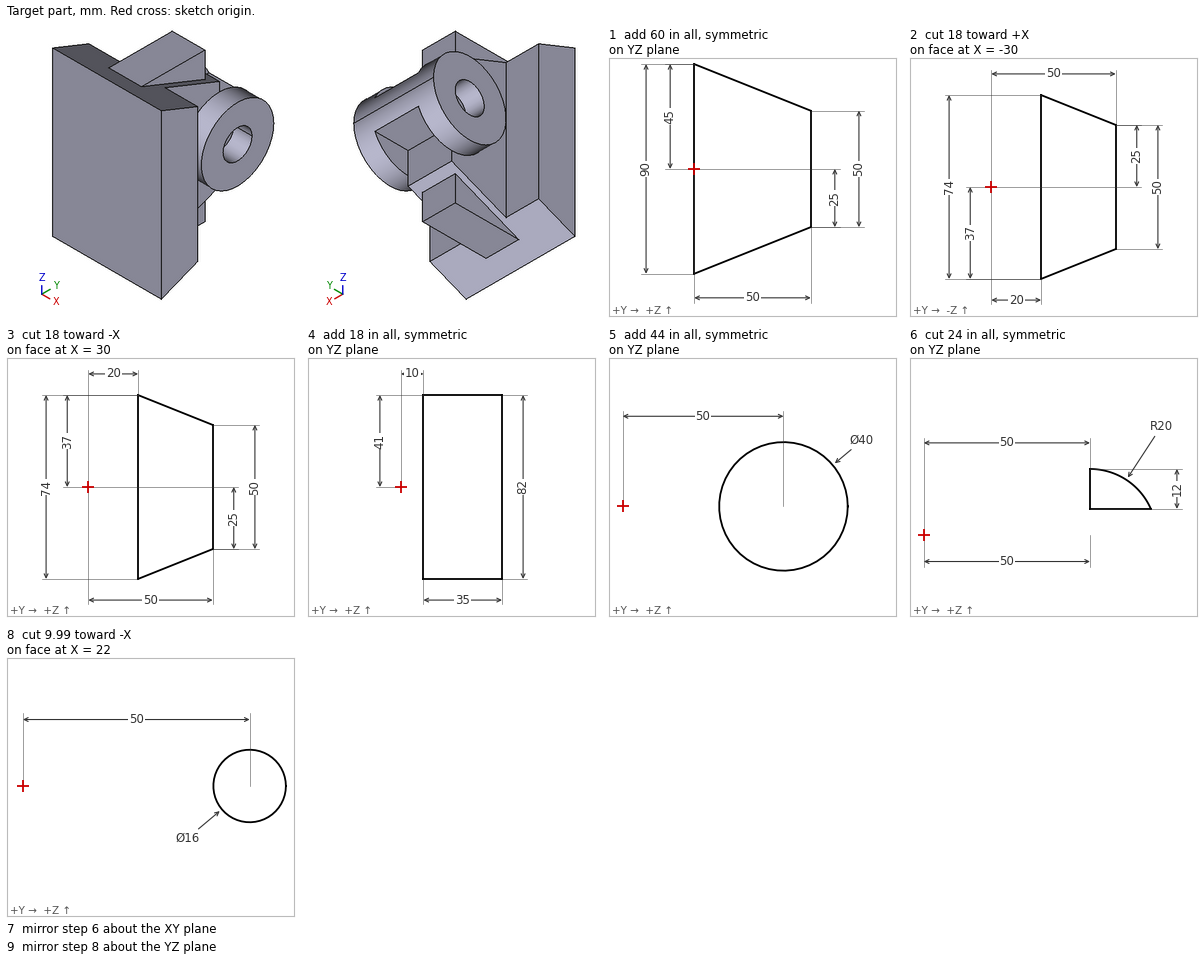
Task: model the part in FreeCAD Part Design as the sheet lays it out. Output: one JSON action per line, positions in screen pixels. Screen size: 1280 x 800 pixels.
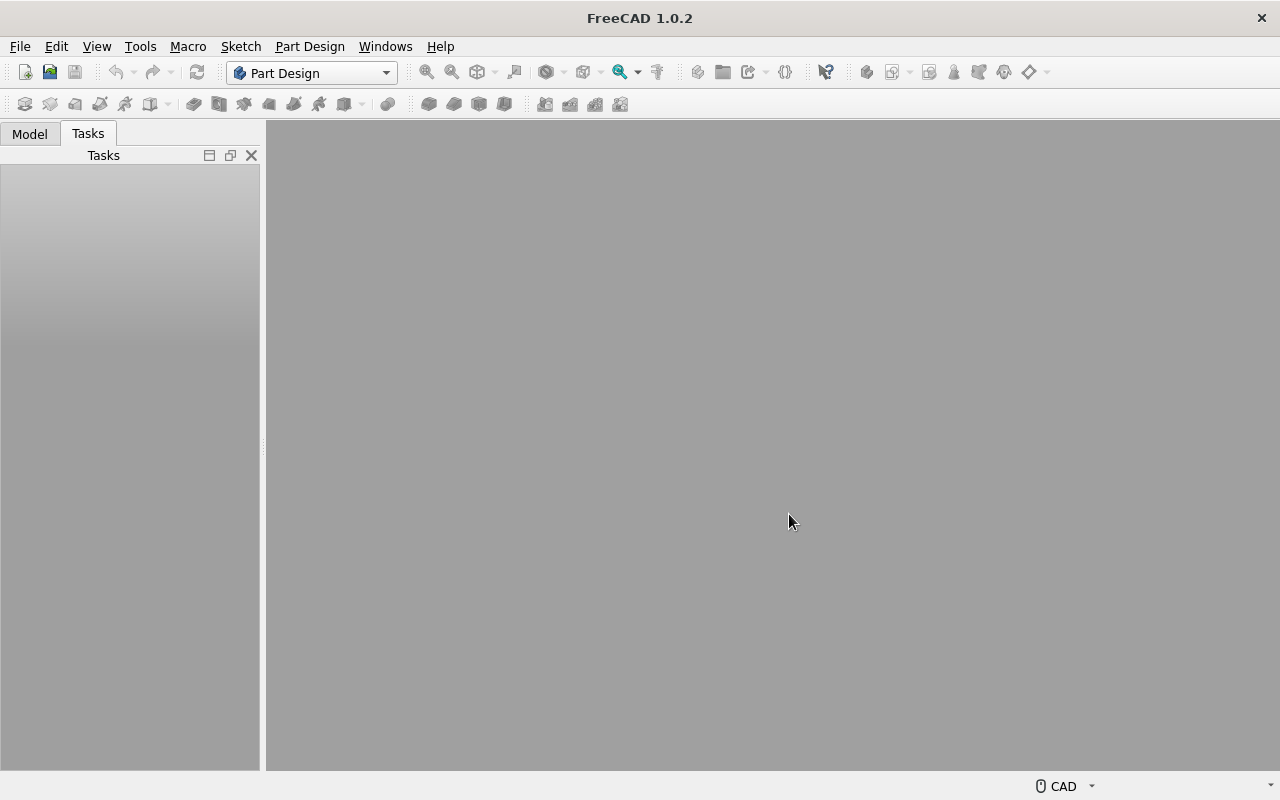
{"action": "left_click", "coordinate": [25, 72]}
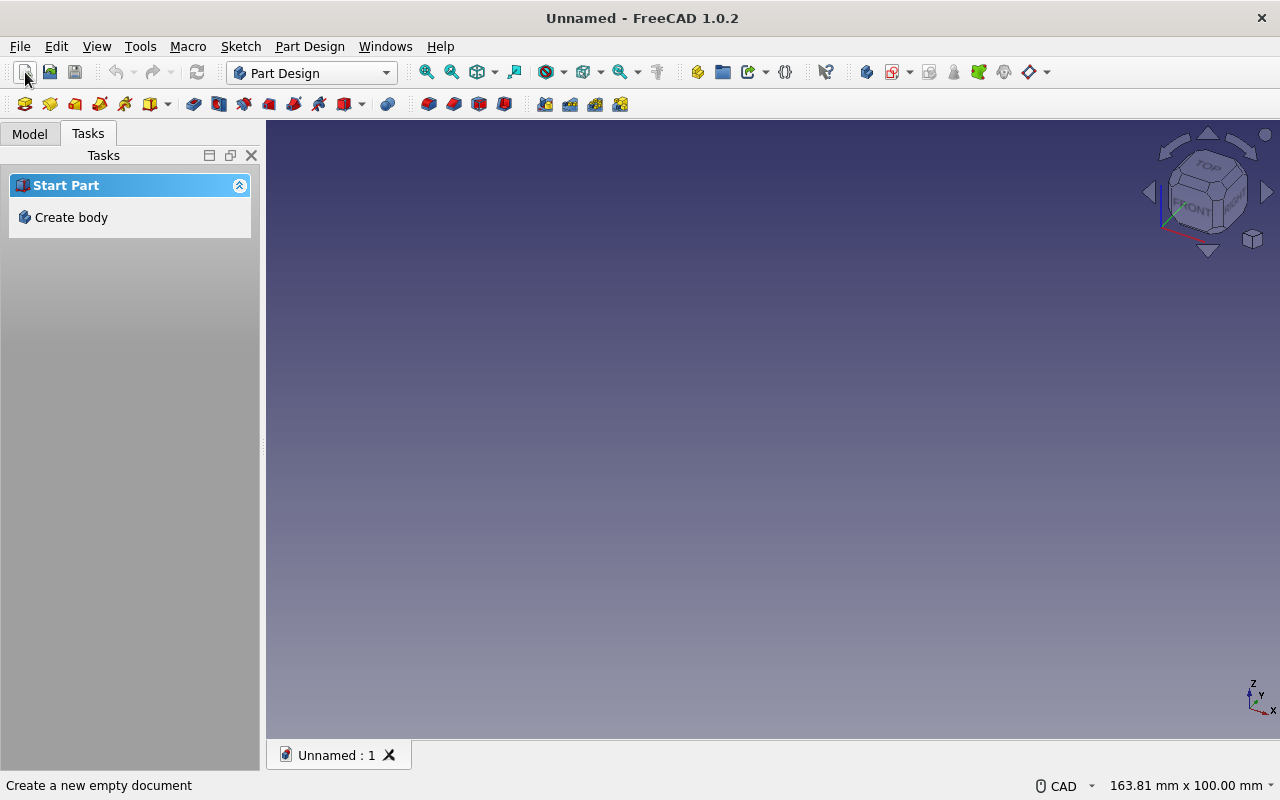
{"action": "left_click", "coordinate": [892, 72]}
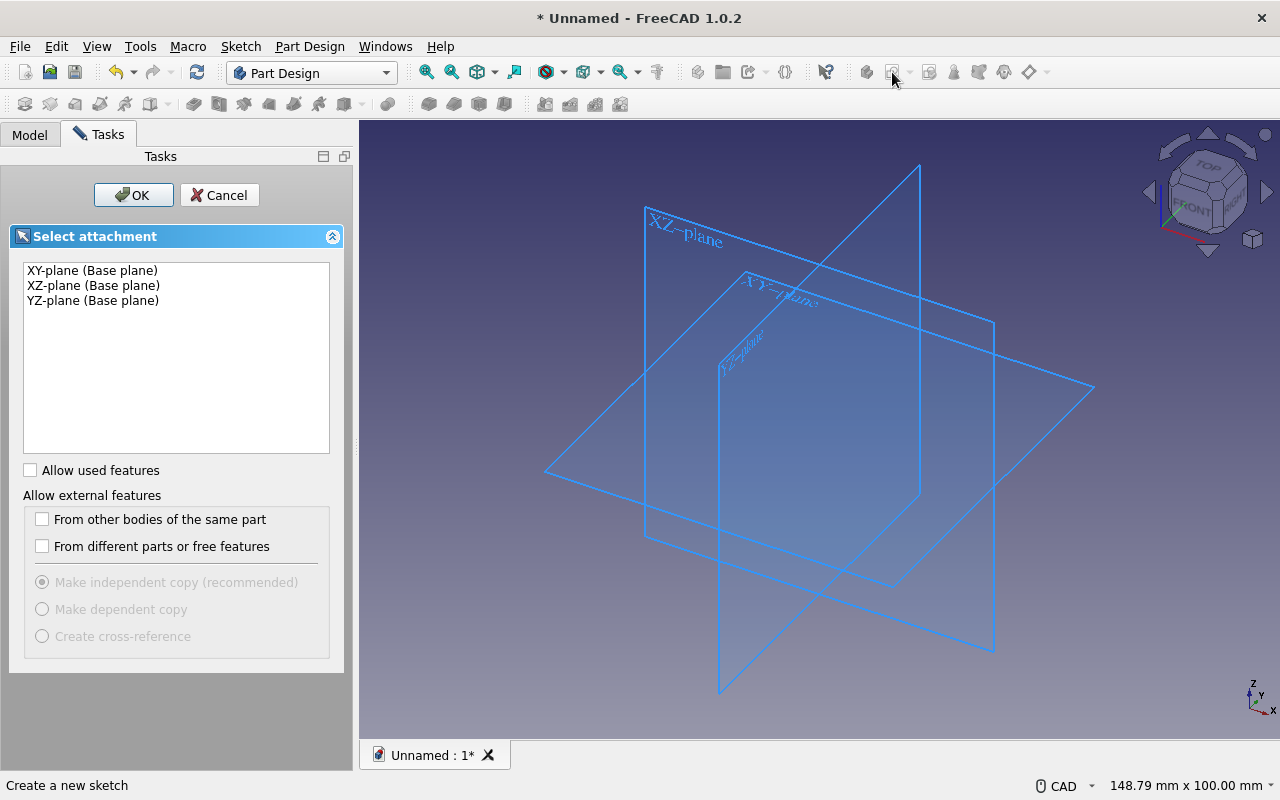
{"action": "left_click", "coordinate": [84, 300]}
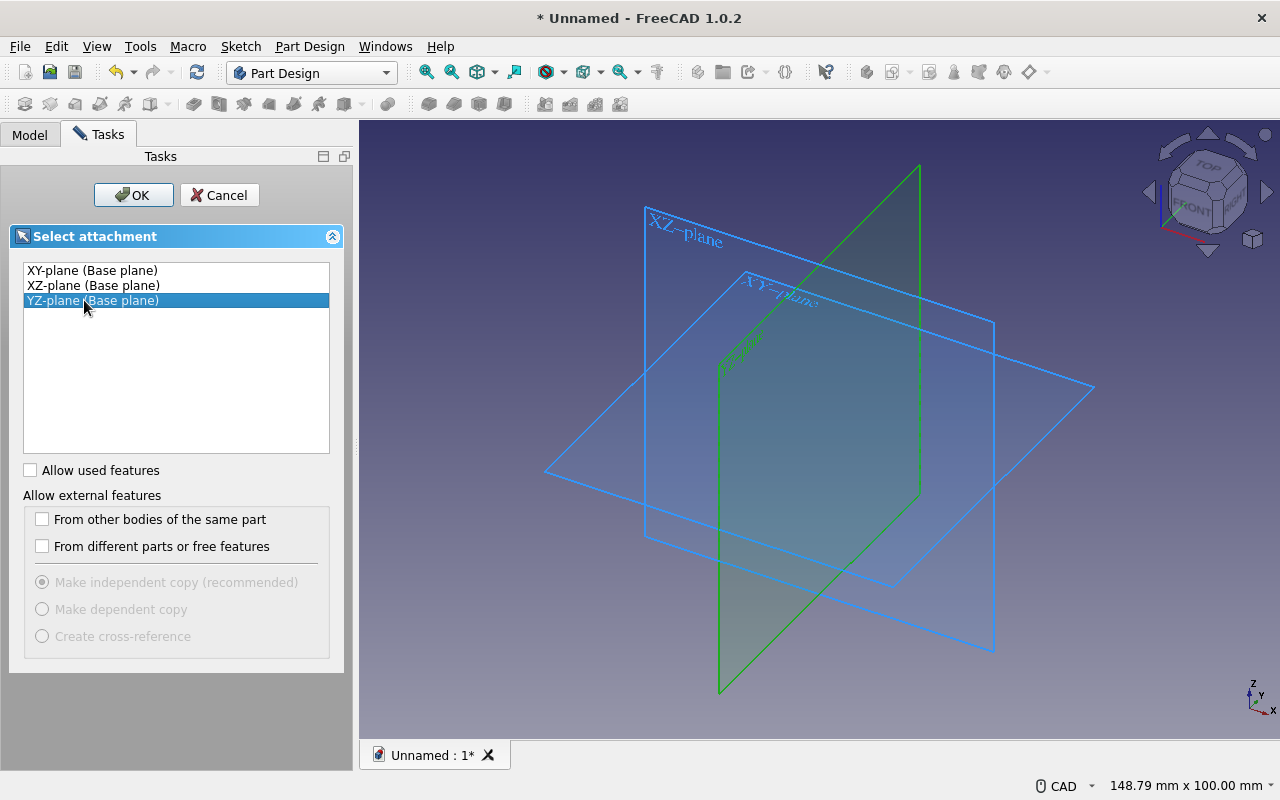
{"action": "left_click", "coordinate": [134, 195]}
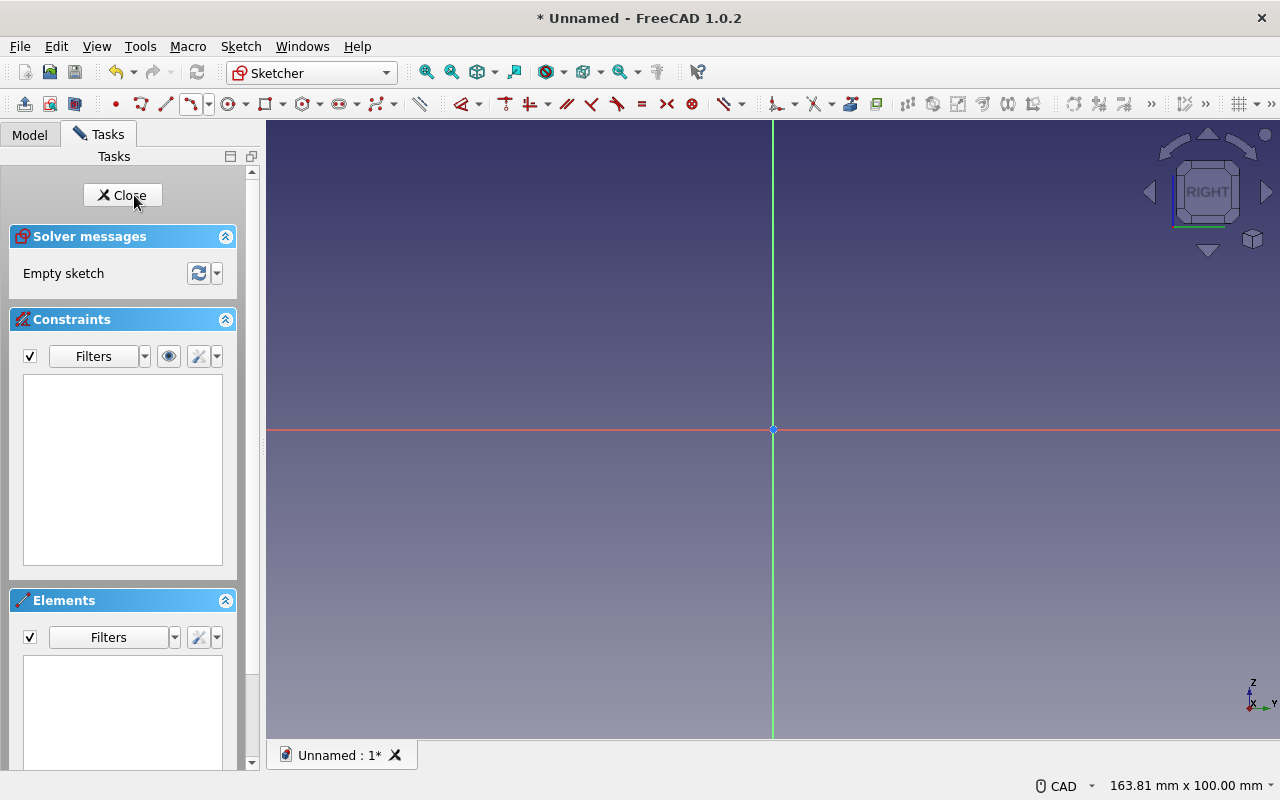
{"action": "scroll", "coordinate": [294, 429], "scroll_direction": "down", "scroll_amount": 2}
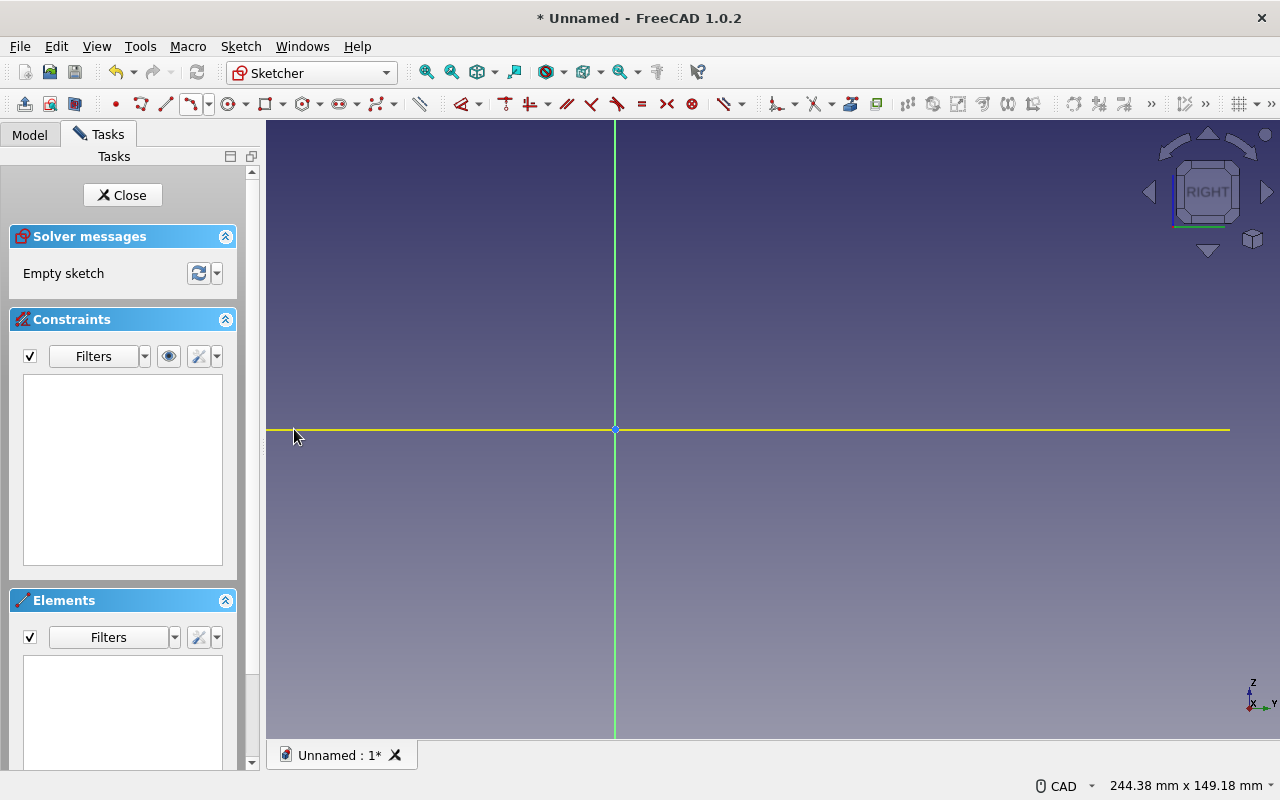
{"action": "left_click", "coordinate": [141, 104]}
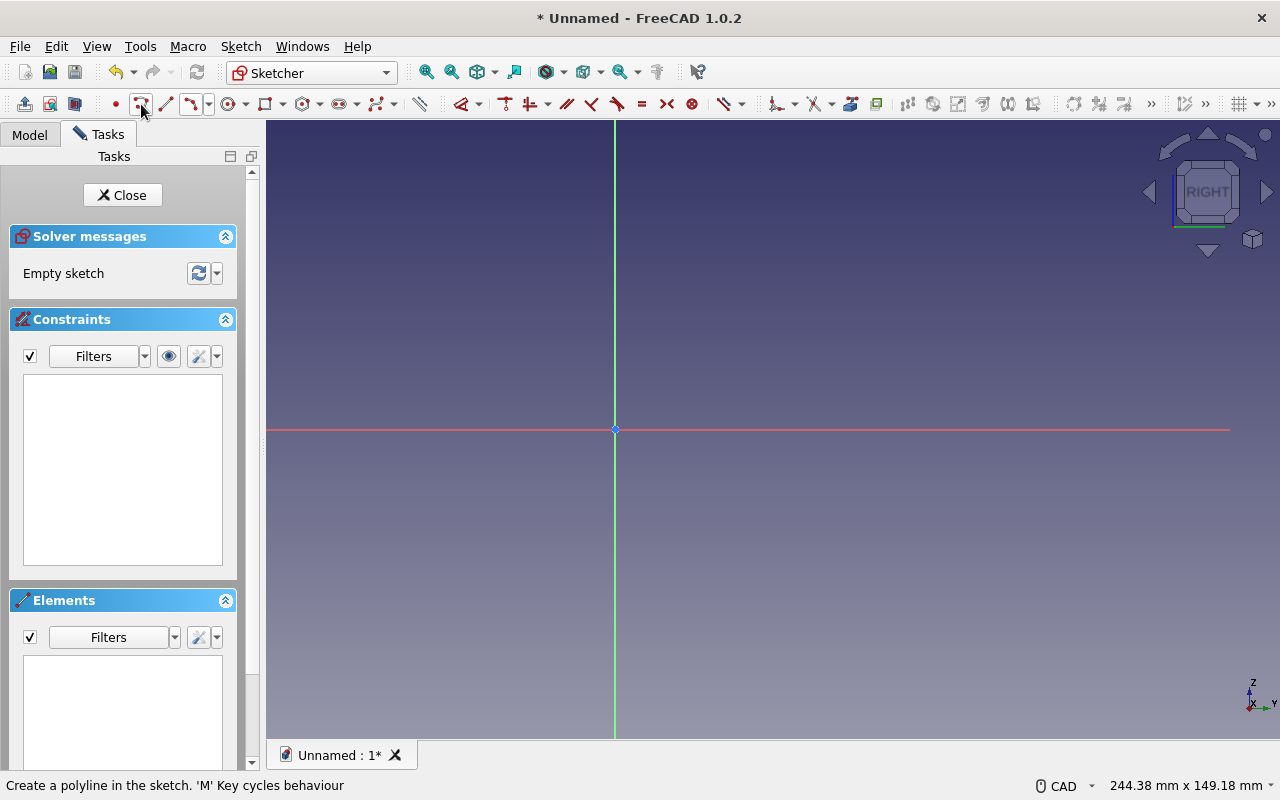
{"action": "left_click", "coordinate": [615, 243]}
{"action": "left_click", "coordinate": [624, 616]}
{"action": "left_click", "coordinate": [823, 533]}
{"action": "left_click", "coordinate": [823, 326]}
{"action": "left_click", "coordinate": [615, 244]}
{"action": "key", "text": "Escape"}
{"action": "key", "text": "Escape"}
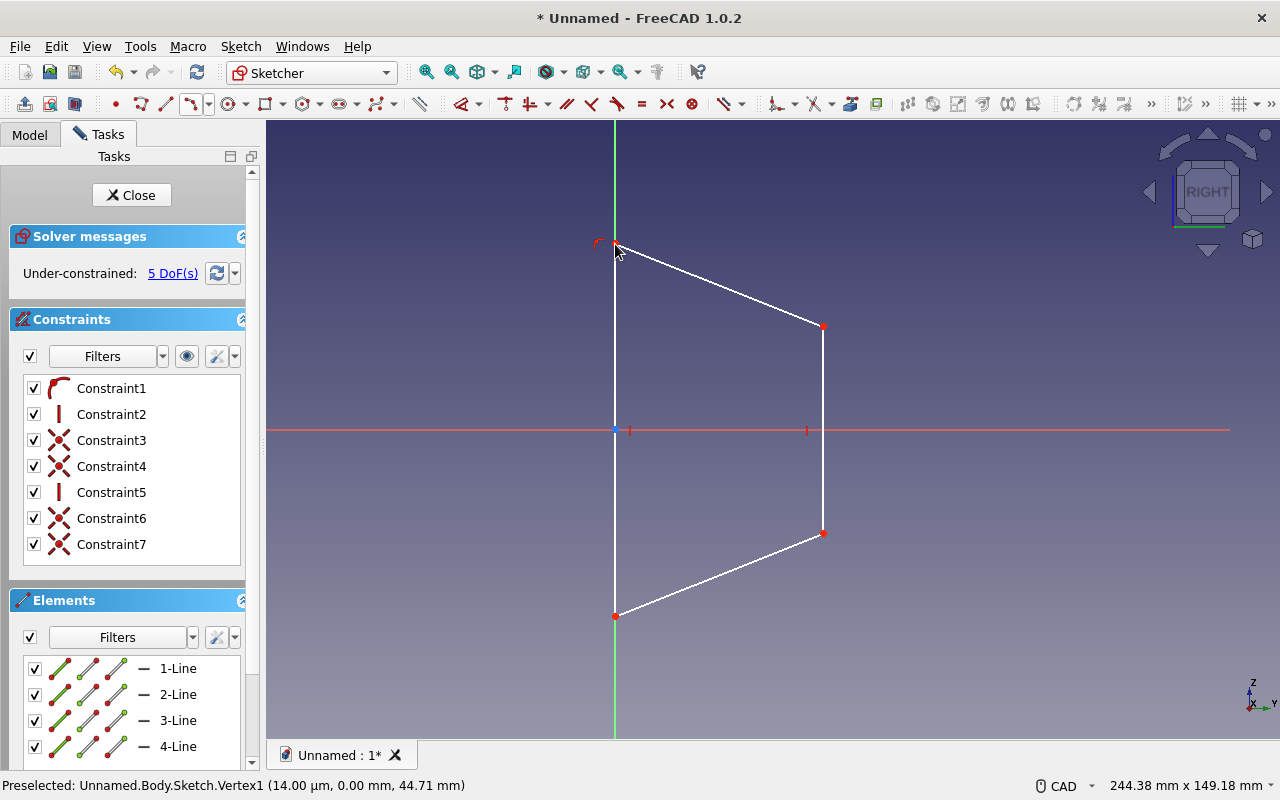
{"action": "left_click", "coordinate": [460, 104]}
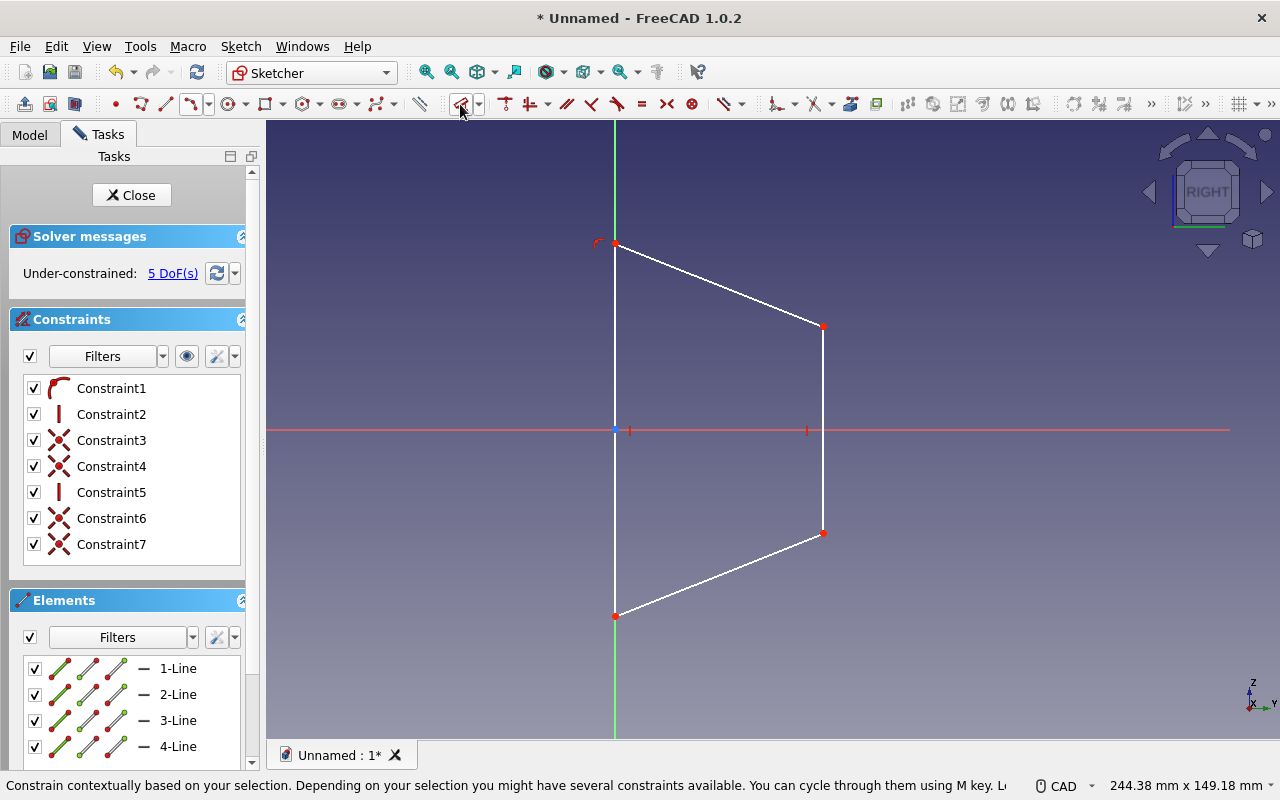
{"action": "left_click", "coordinate": [615, 356]}
{"action": "left_click", "coordinate": [581, 345]}